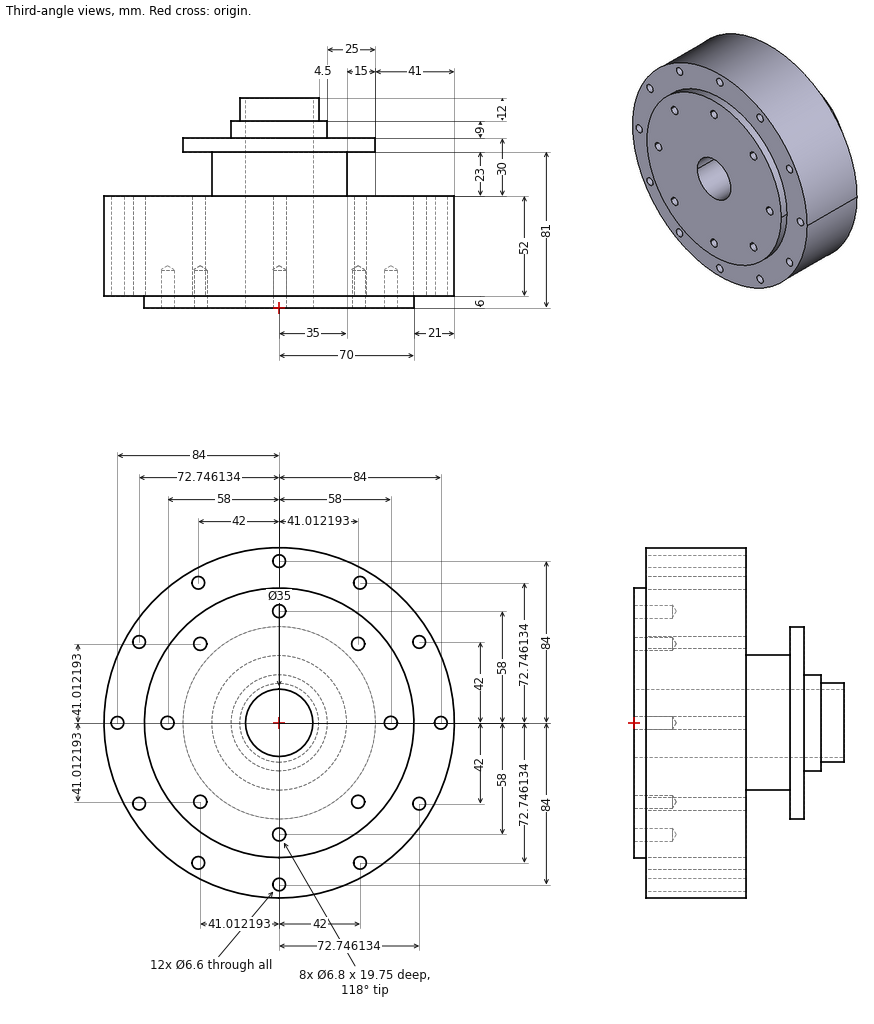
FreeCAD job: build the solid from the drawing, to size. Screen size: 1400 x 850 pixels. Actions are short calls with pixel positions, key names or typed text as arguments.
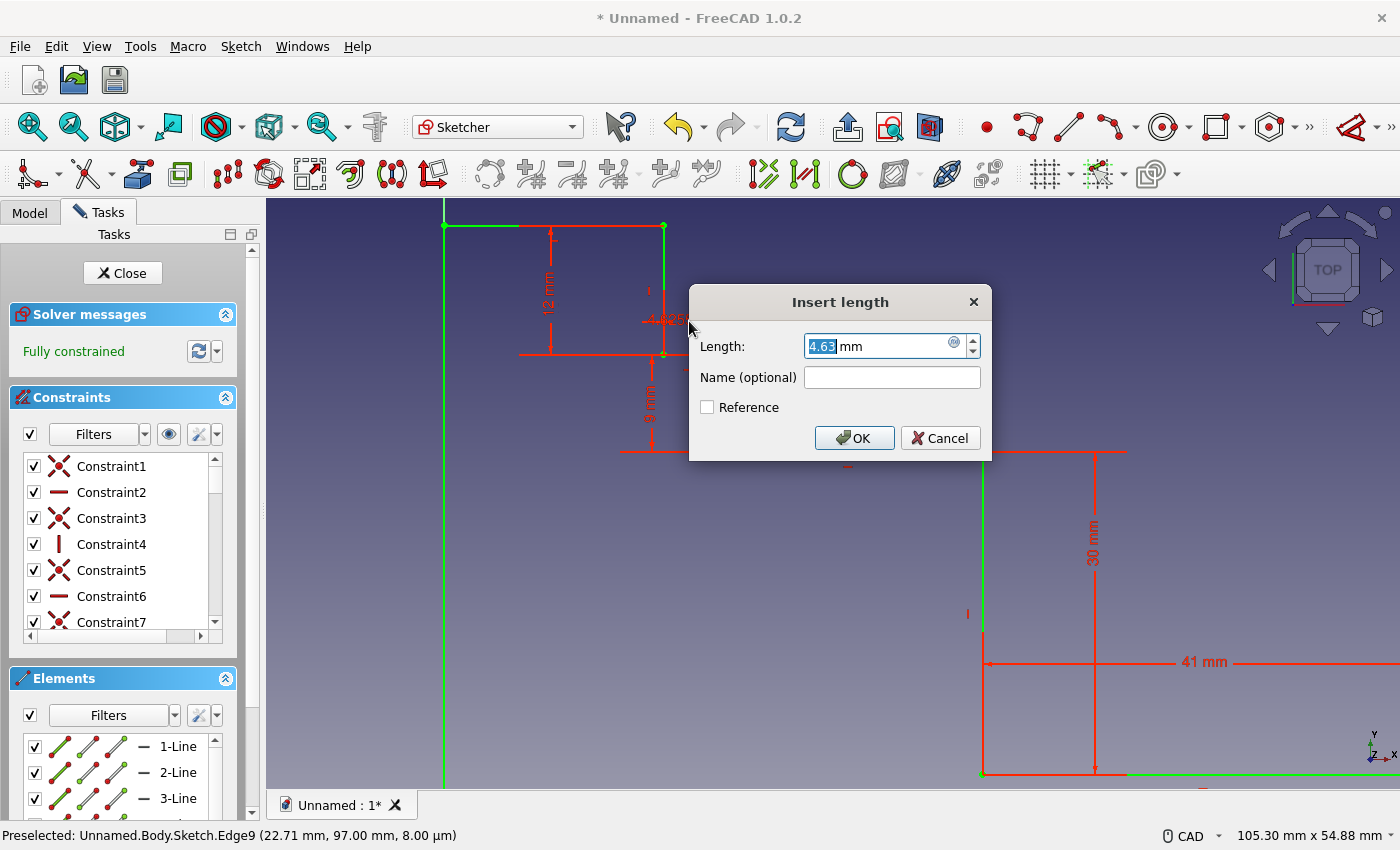
text(4.5)
key(Return)
key(Escape)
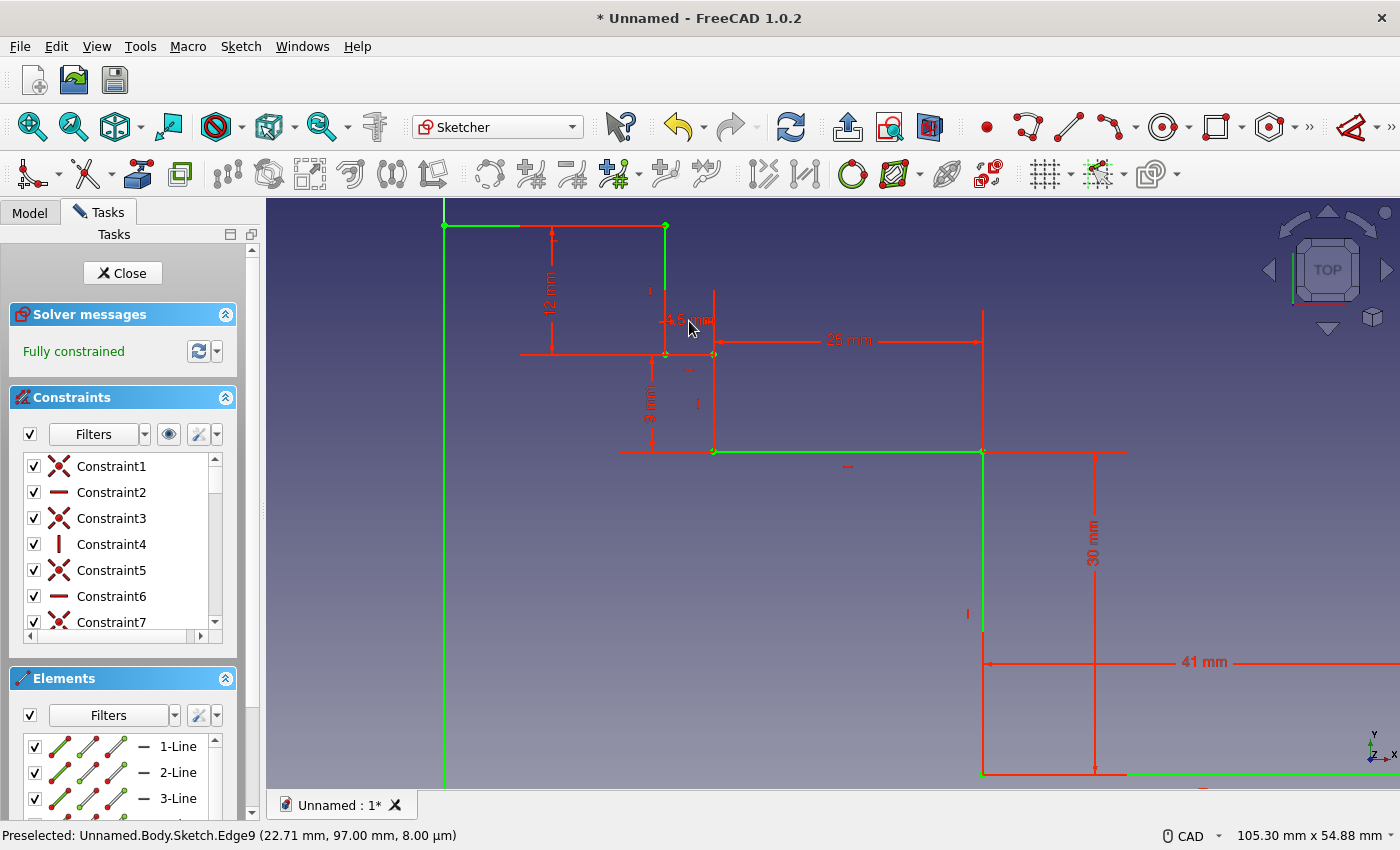
click(123, 273)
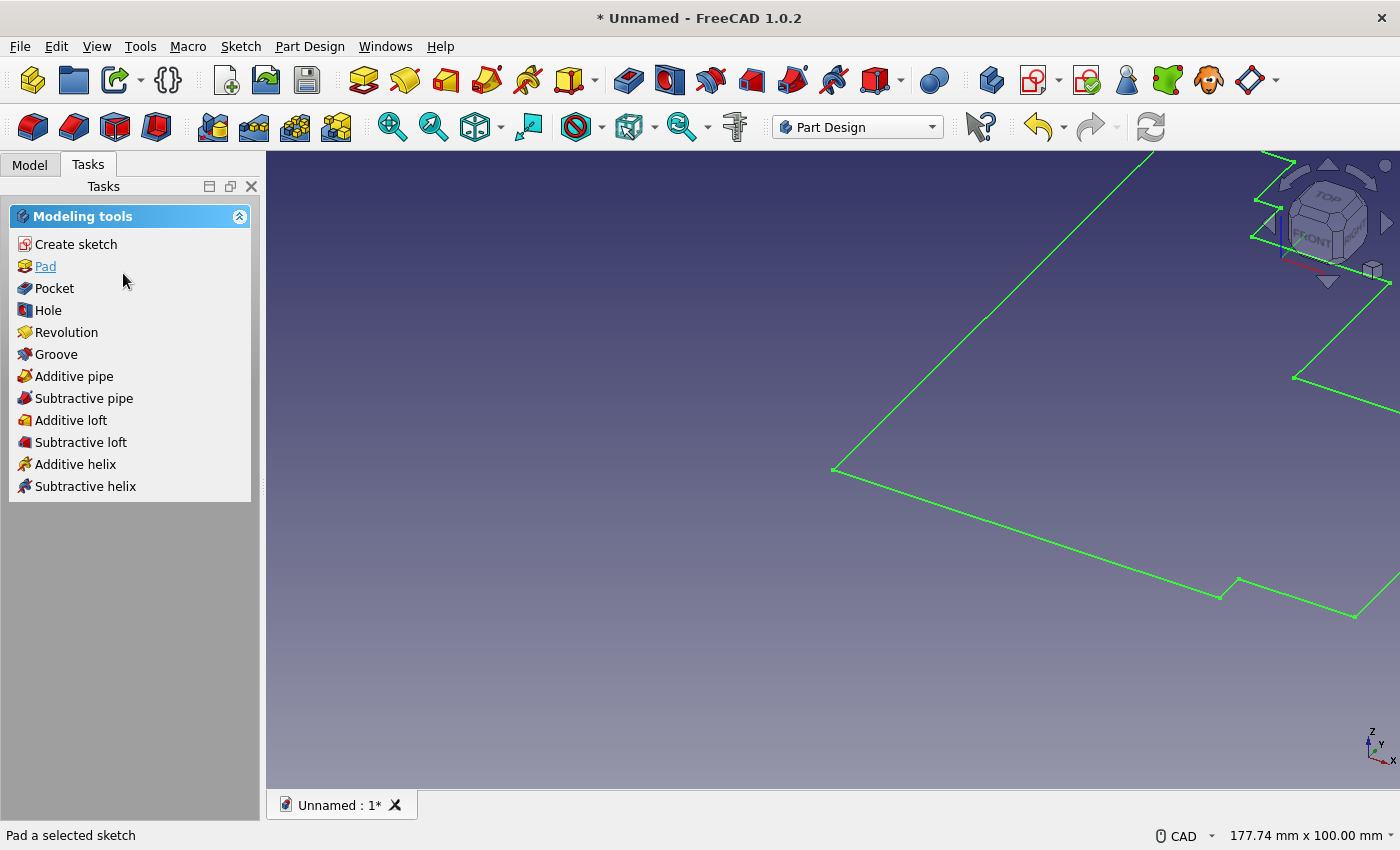
click(405, 80)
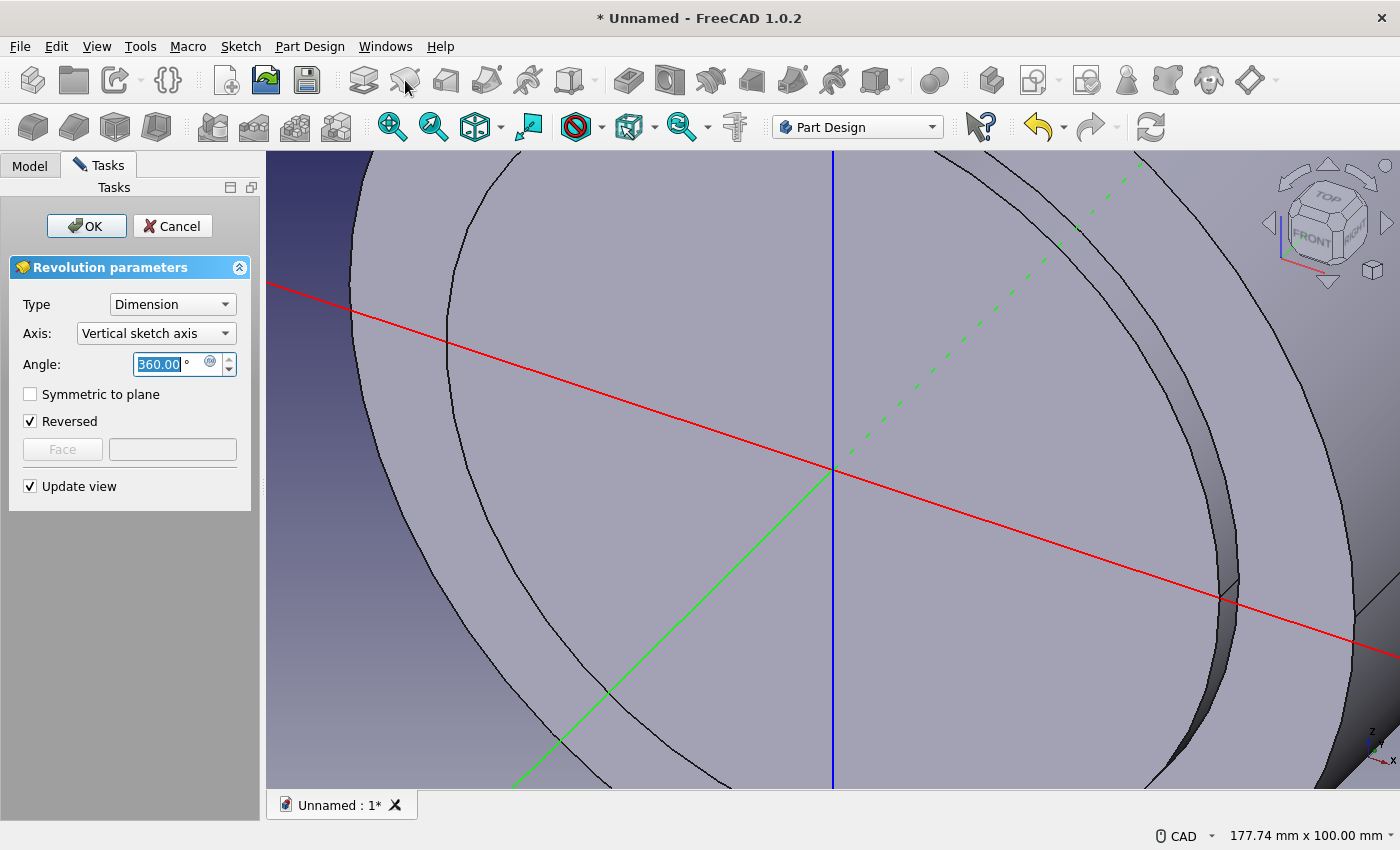
click(87, 226)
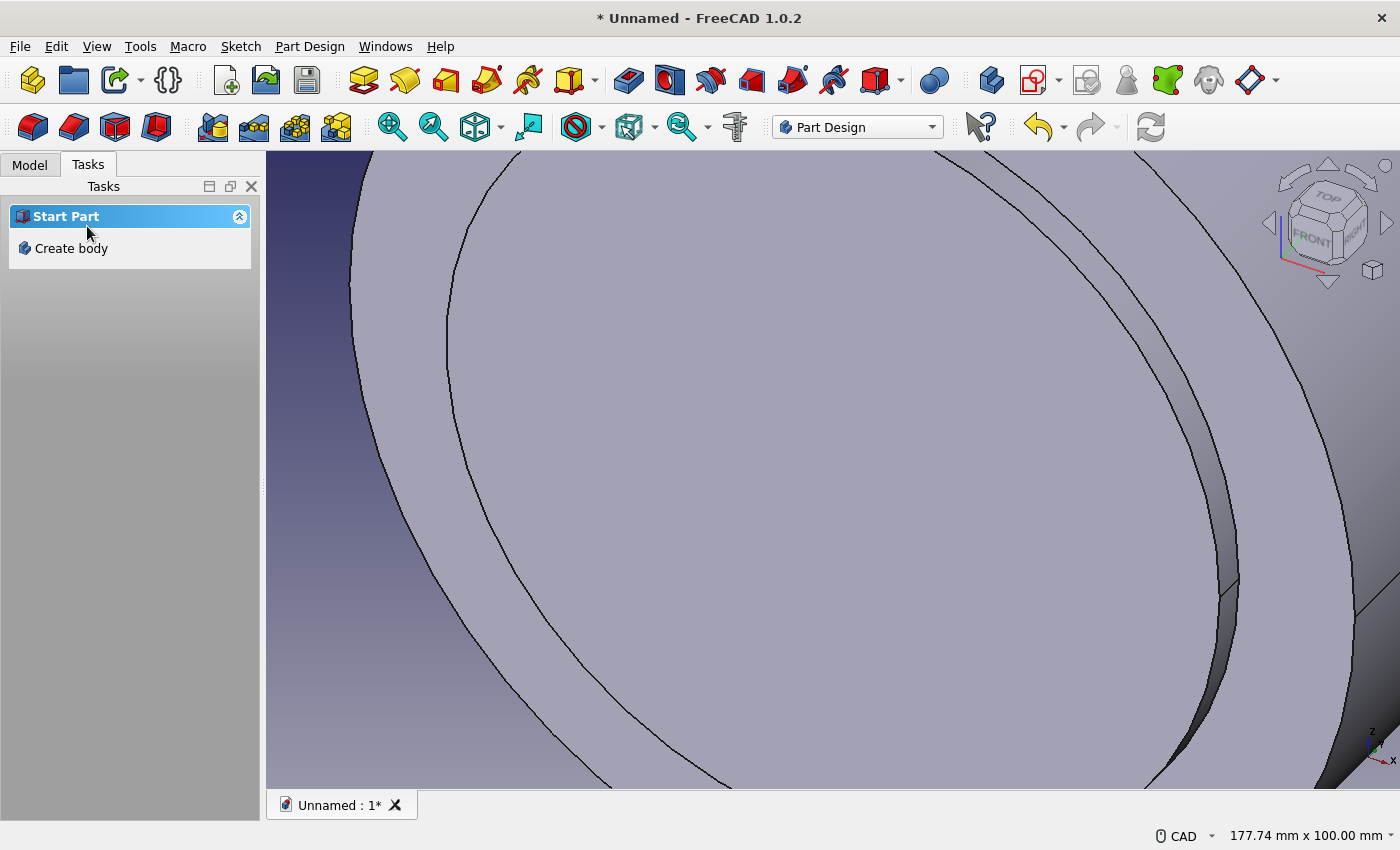
click(393, 128)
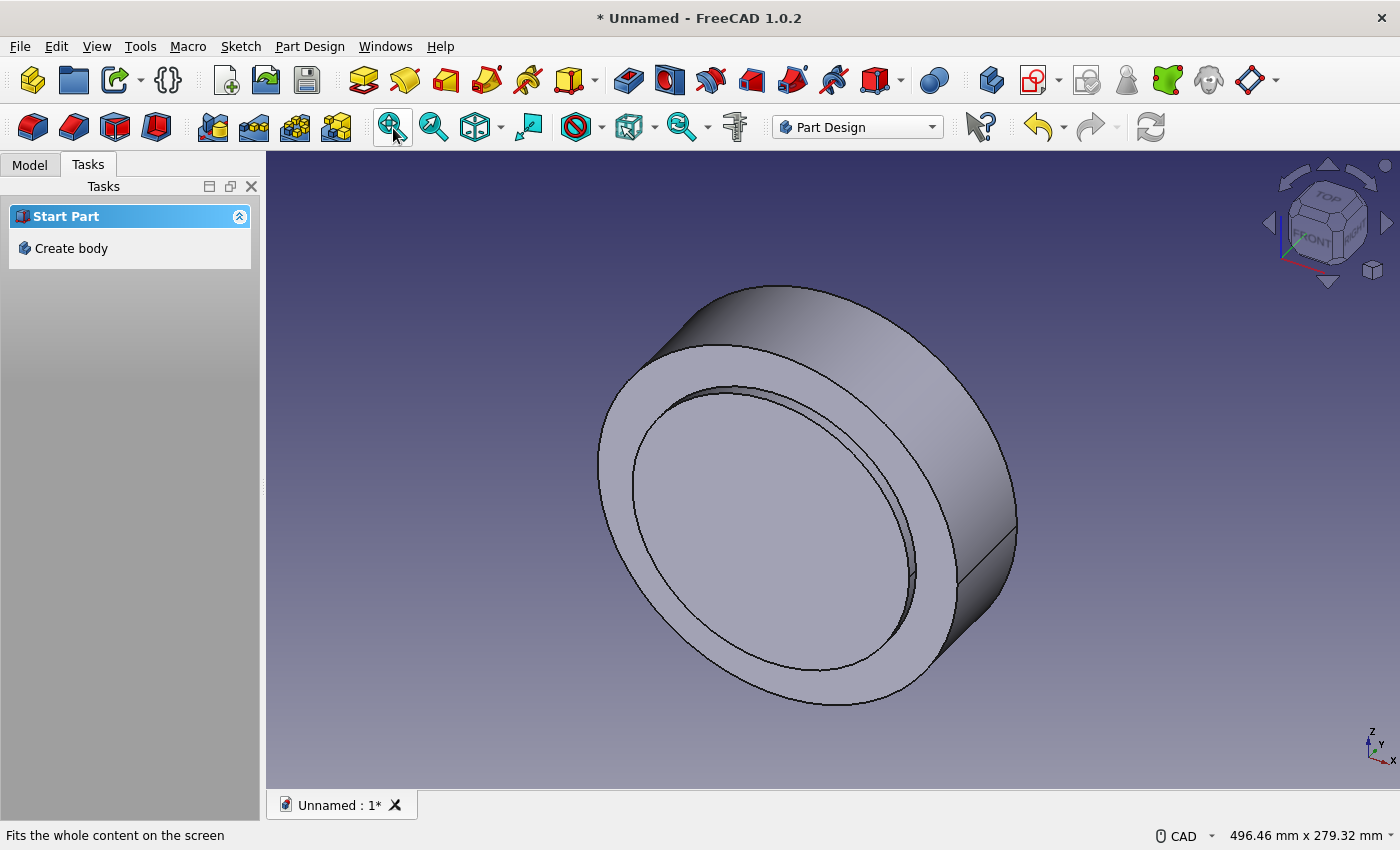
key(4)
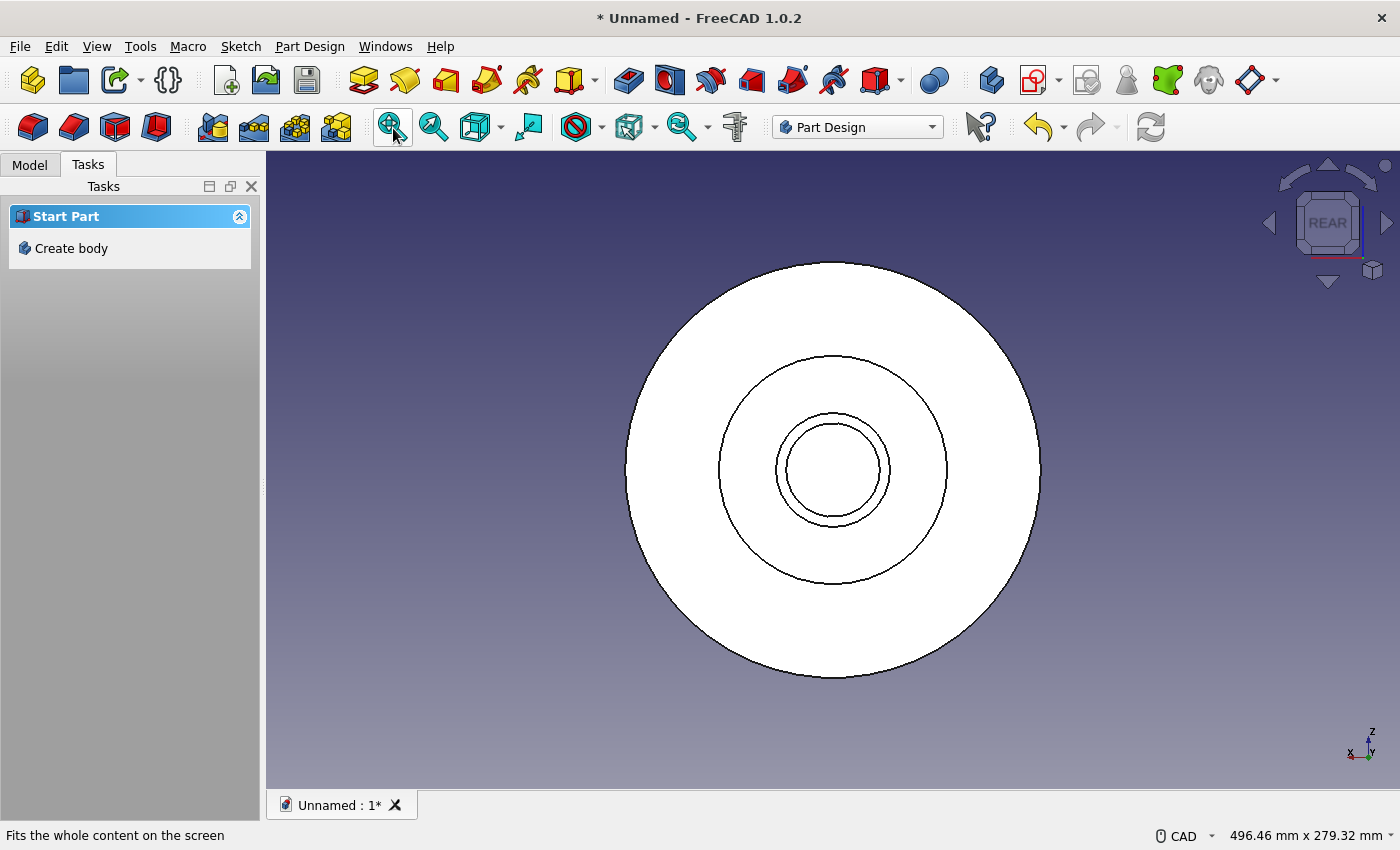
click(833, 469)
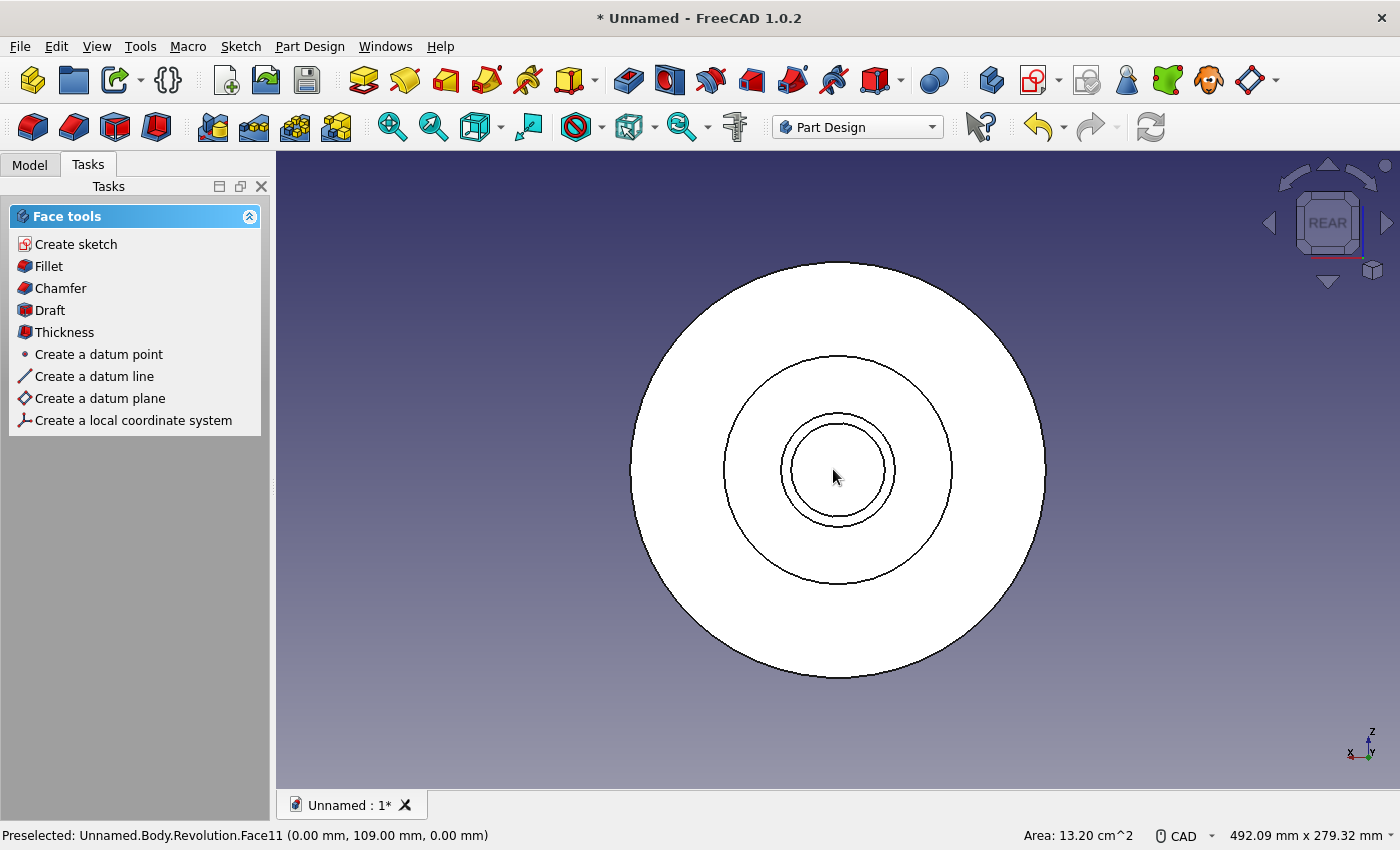
click(1032, 80)